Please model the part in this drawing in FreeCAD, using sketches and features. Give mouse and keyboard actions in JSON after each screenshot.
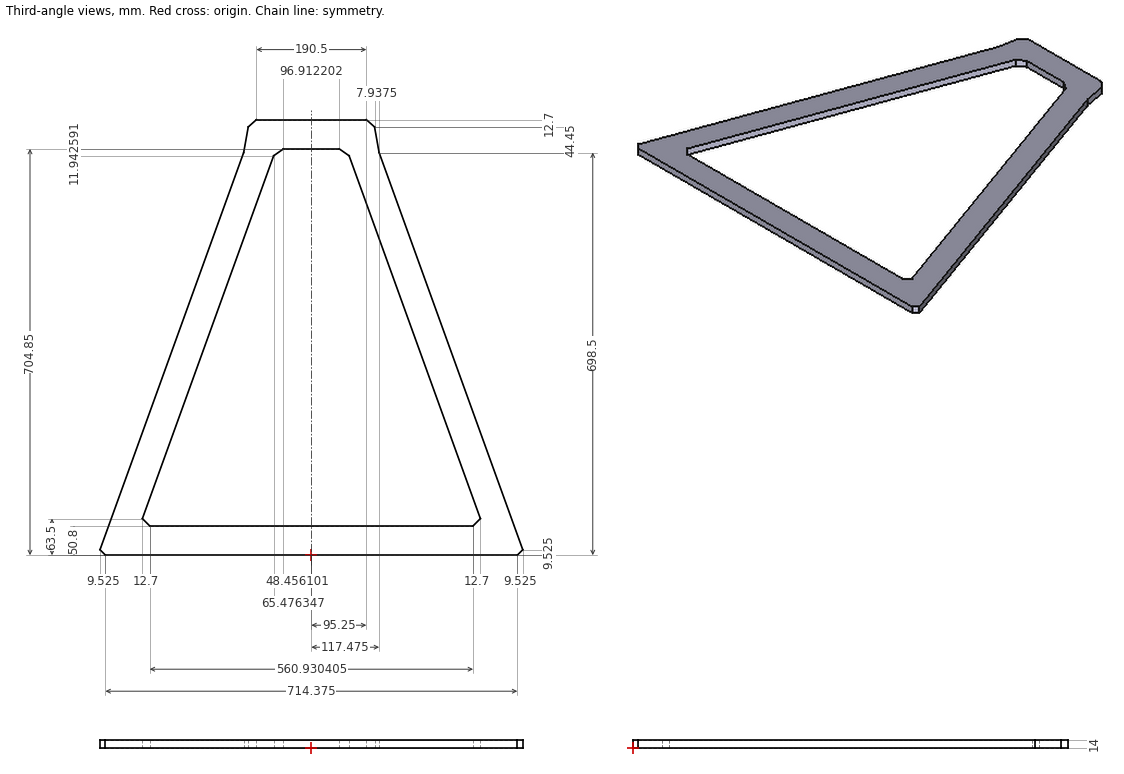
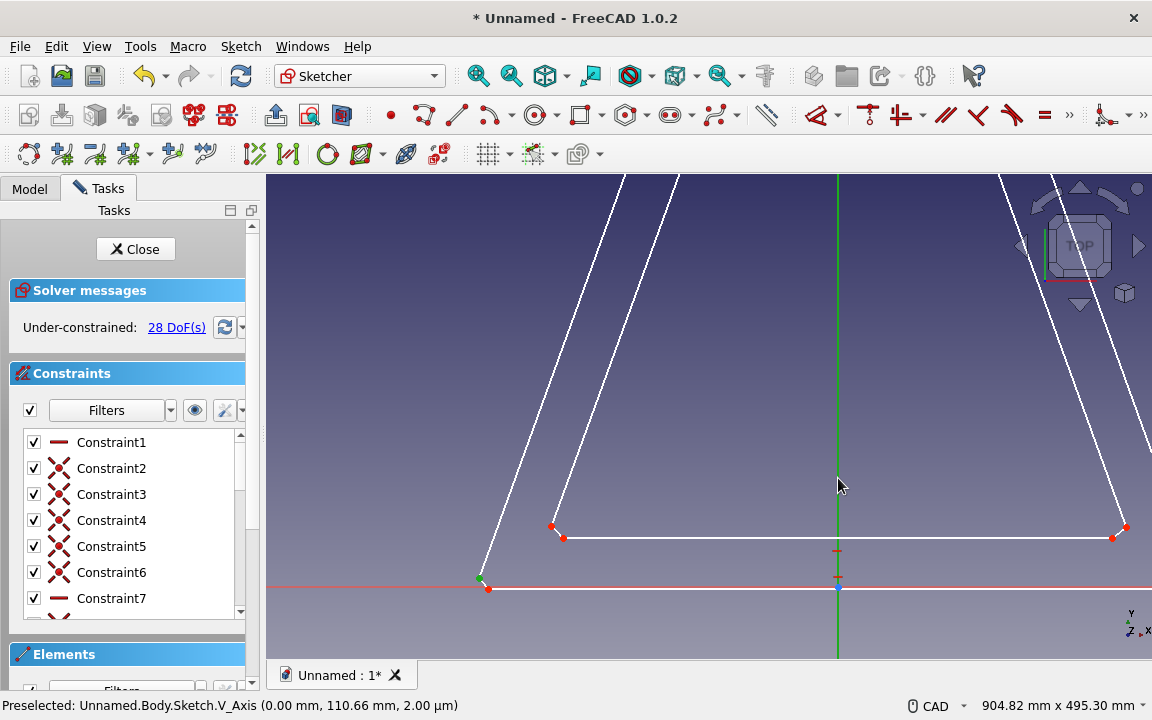
{"action": "key", "text": "s"}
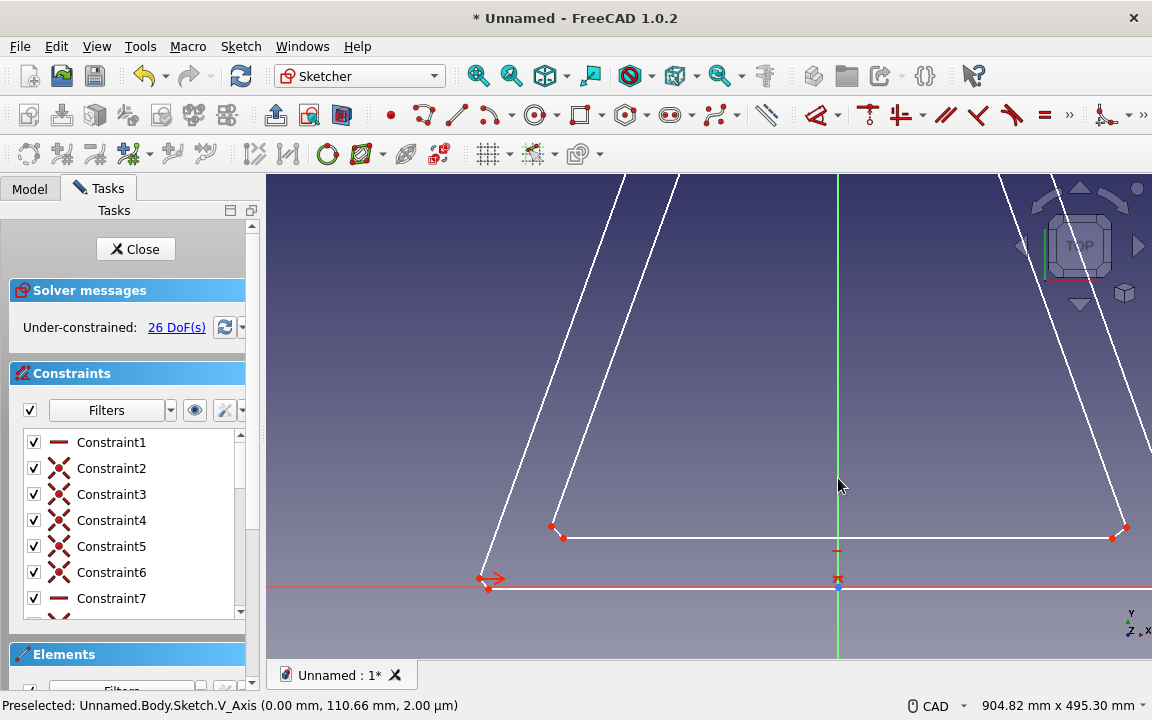
{"action": "scroll", "coordinate": [479, 579], "scroll_direction": "down", "scroll_amount": 4}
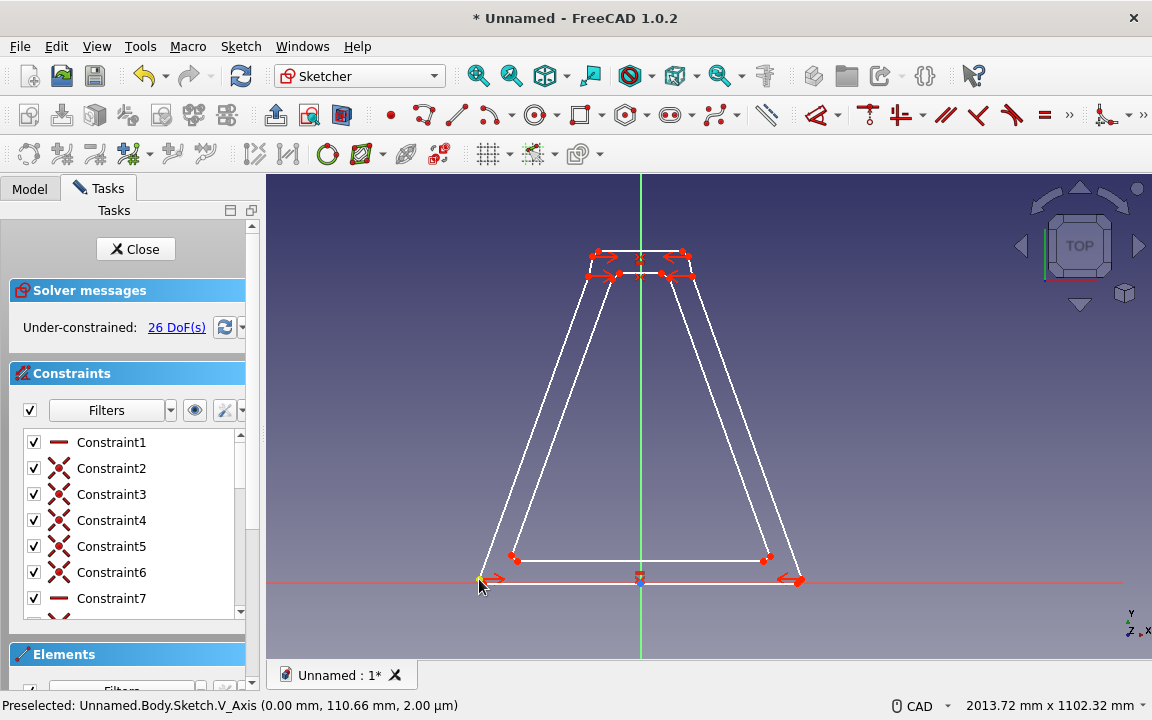
{"action": "scroll", "coordinate": [612, 280], "scroll_direction": "up", "scroll_amount": 2}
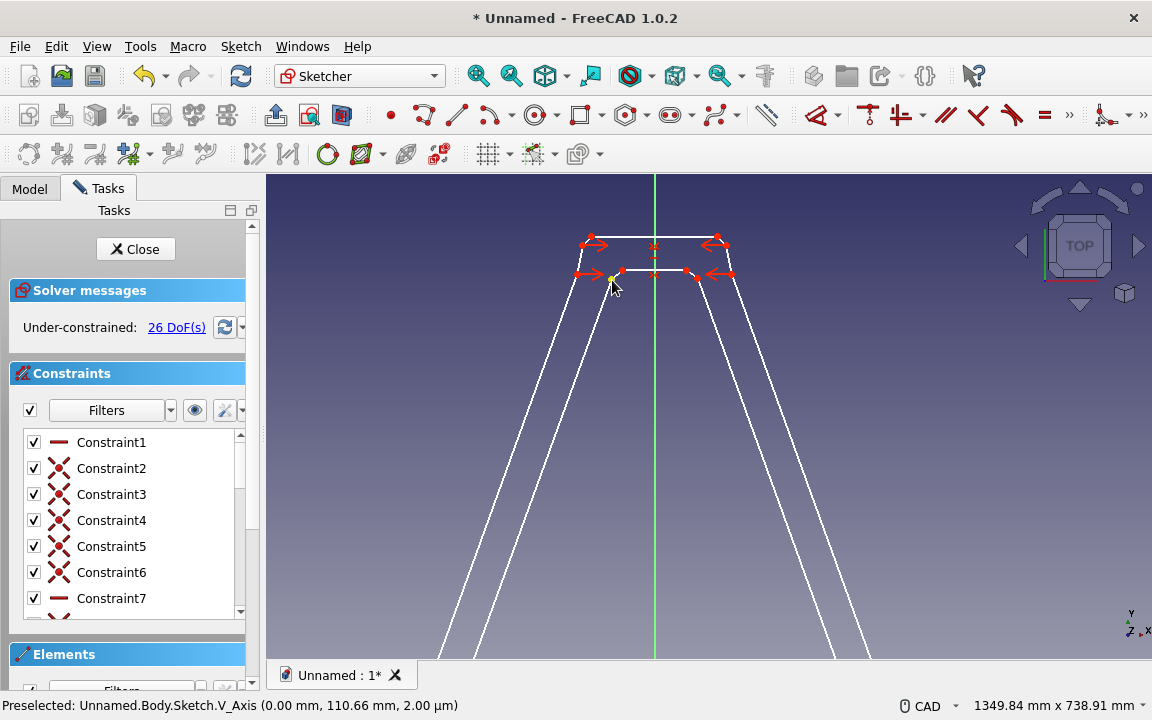
{"action": "left_click", "coordinate": [612, 280]}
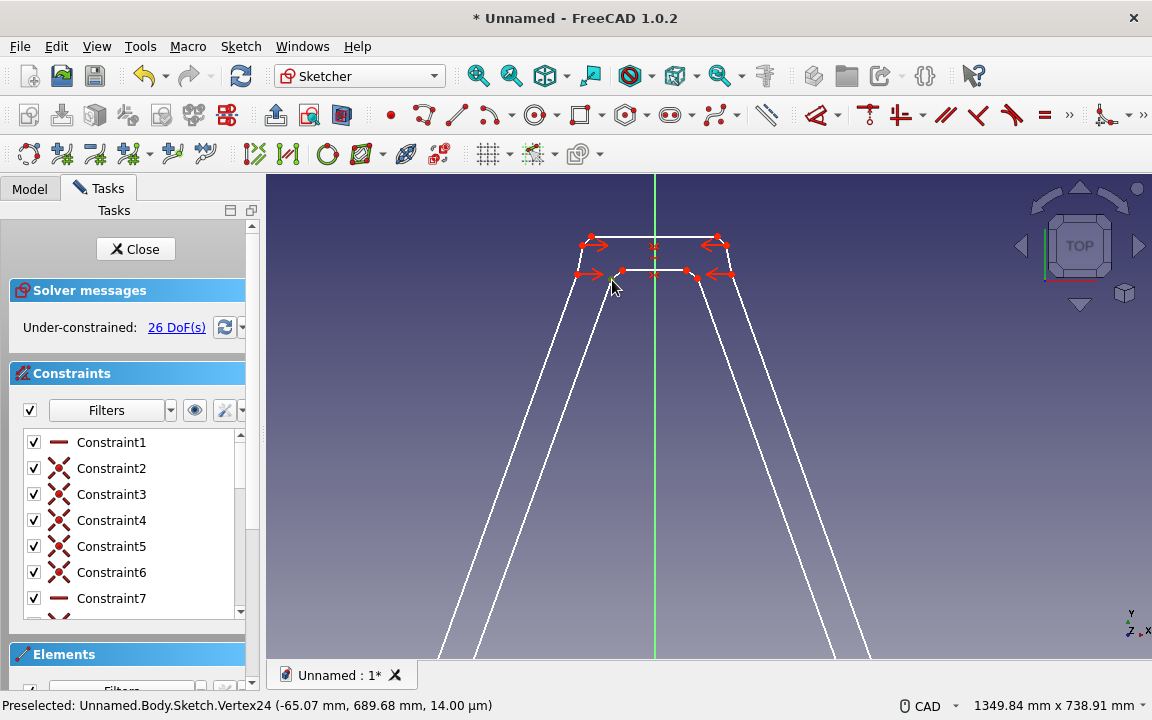
{"action": "left_click", "coordinate": [698, 278]}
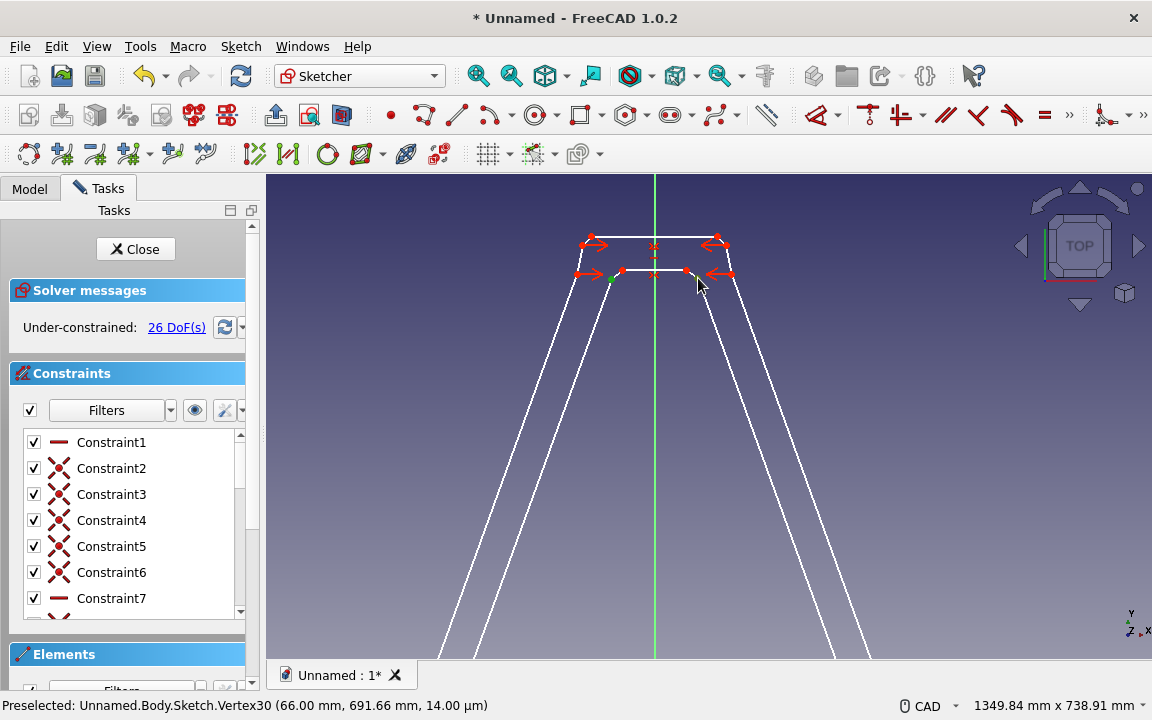
{"action": "left_click", "coordinate": [655, 600]}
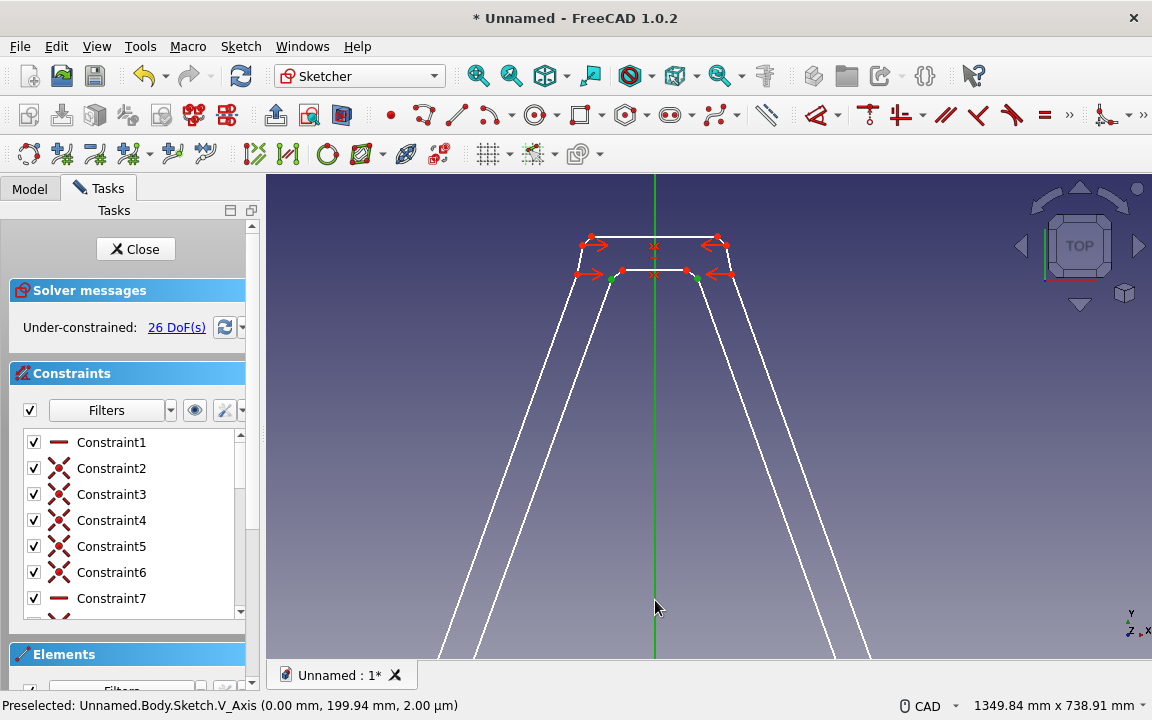
{"action": "key", "text": "s"}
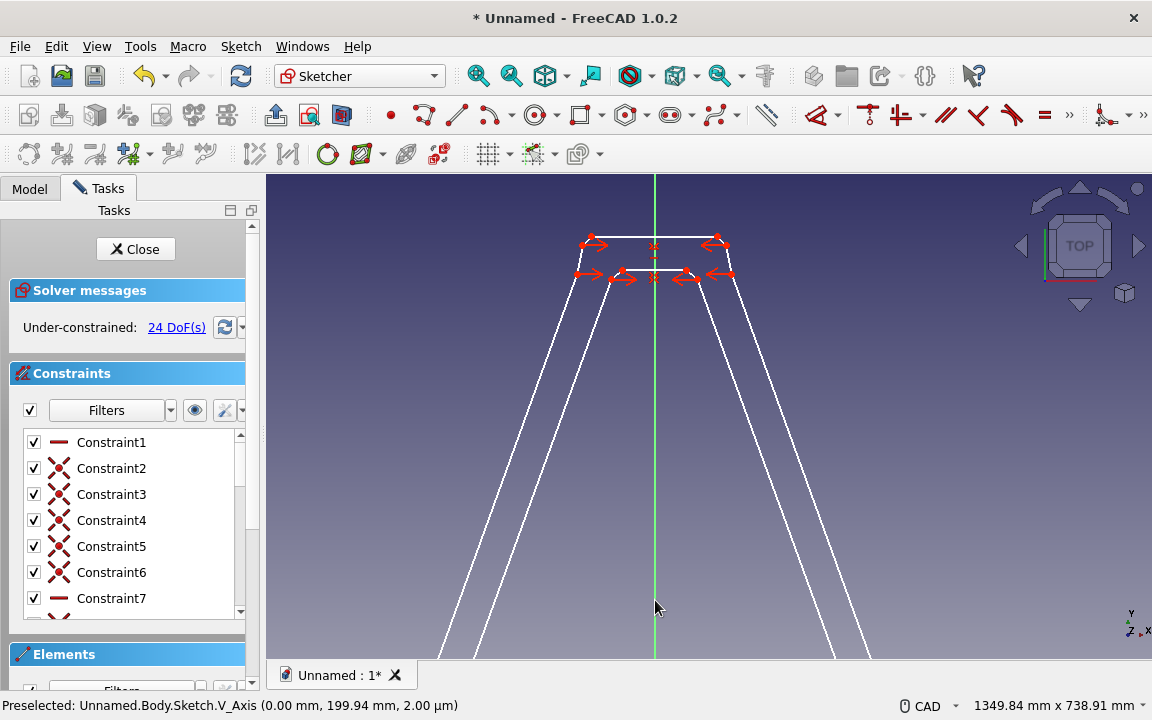
{"action": "scroll", "coordinate": [612, 279], "scroll_direction": "down", "scroll_amount": 2}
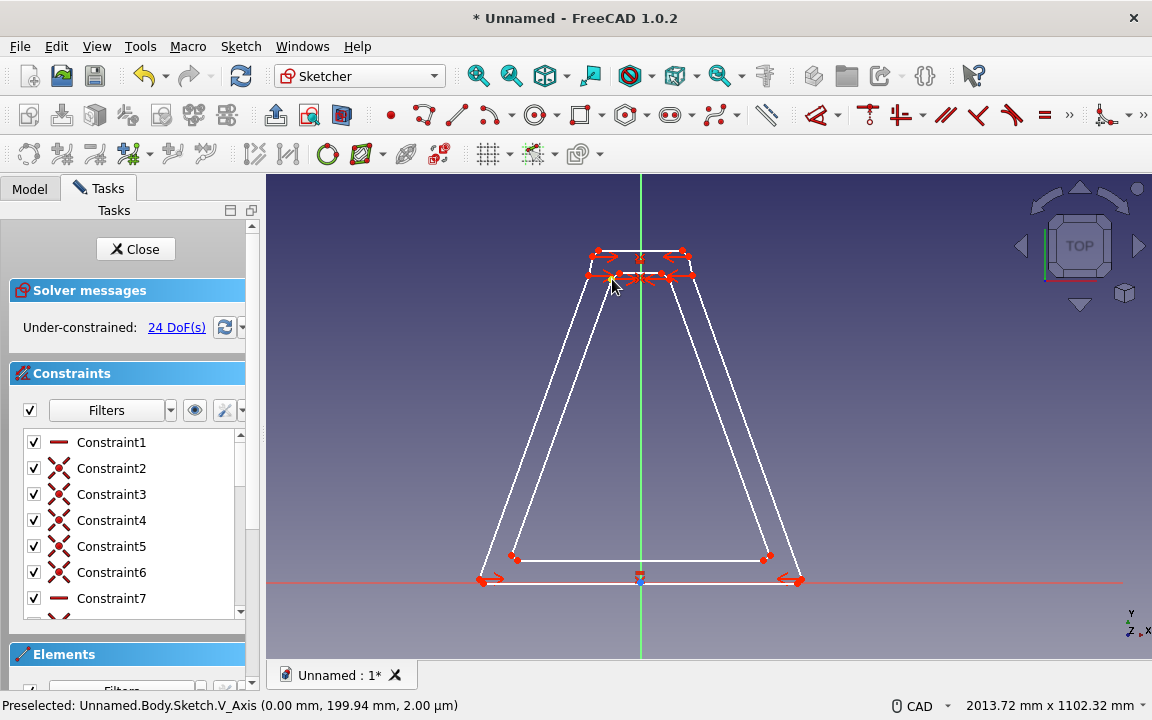
{"action": "scroll", "coordinate": [512, 555], "scroll_direction": "up", "scroll_amount": 3}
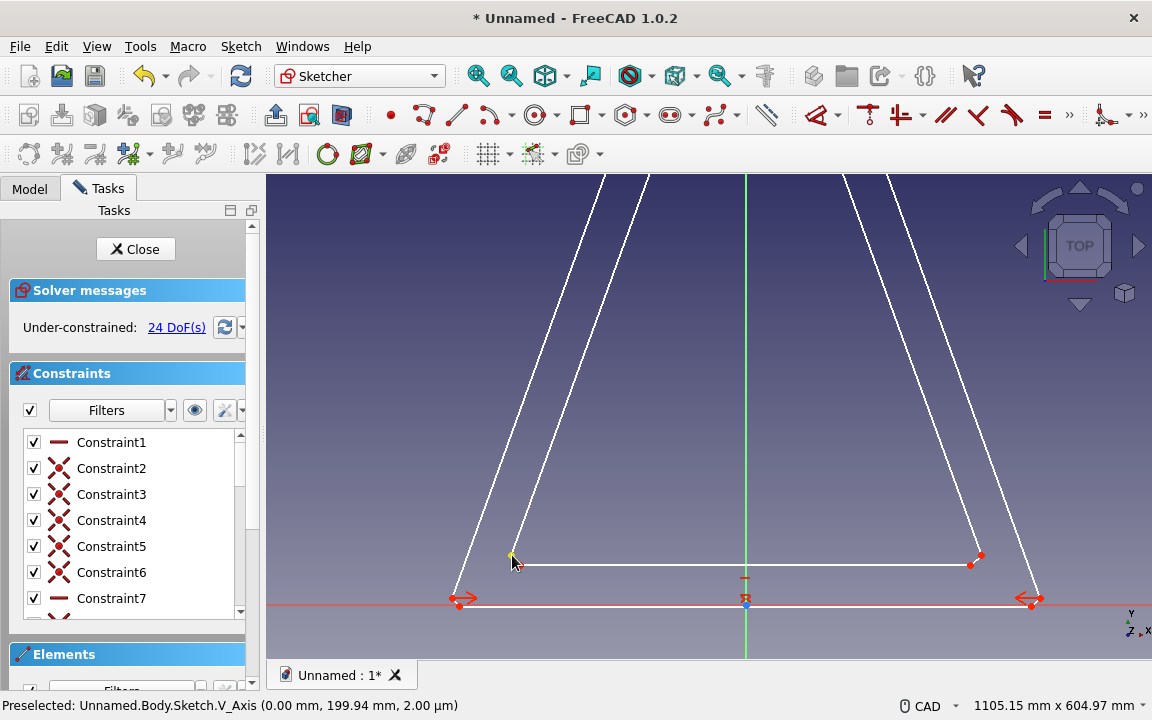
{"action": "left_click", "coordinate": [511, 555]}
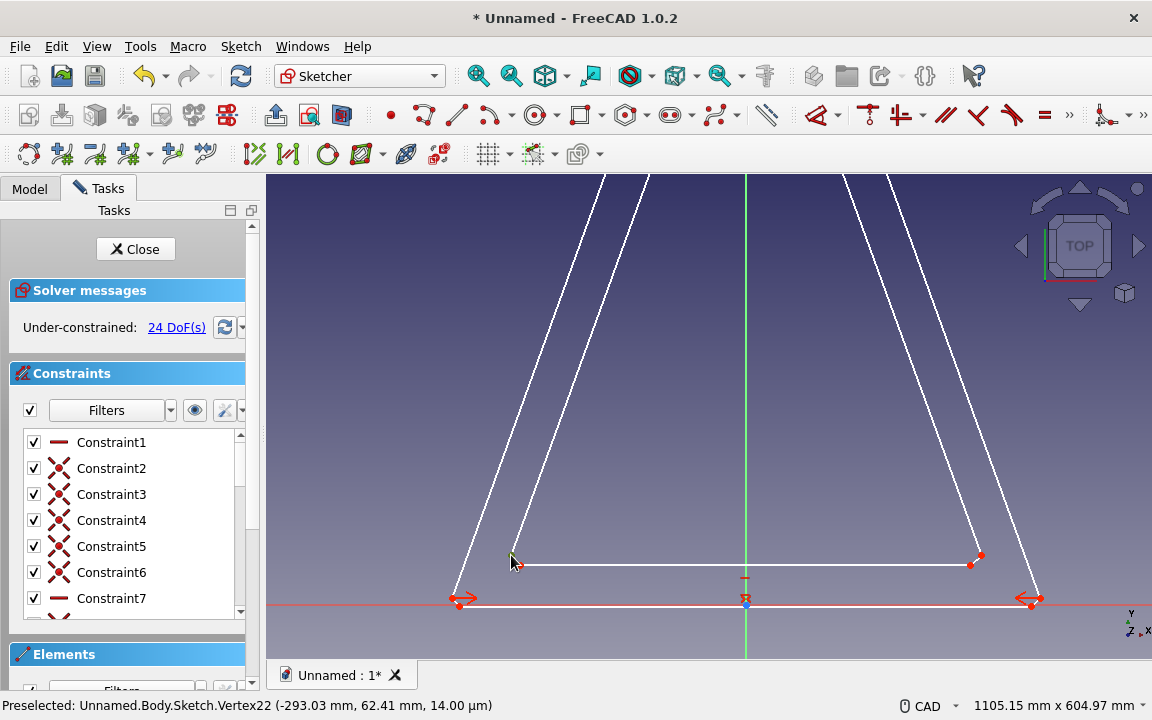
{"action": "left_click", "coordinate": [982, 556]}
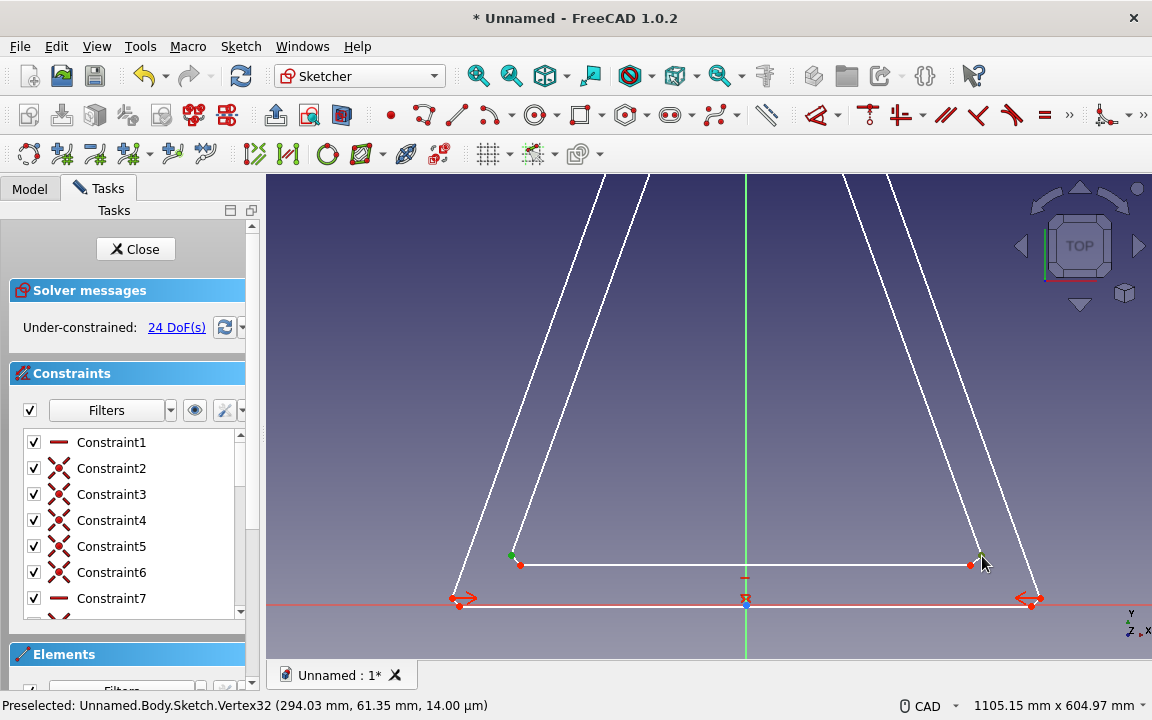
{"action": "left_click", "coordinate": [746, 508]}